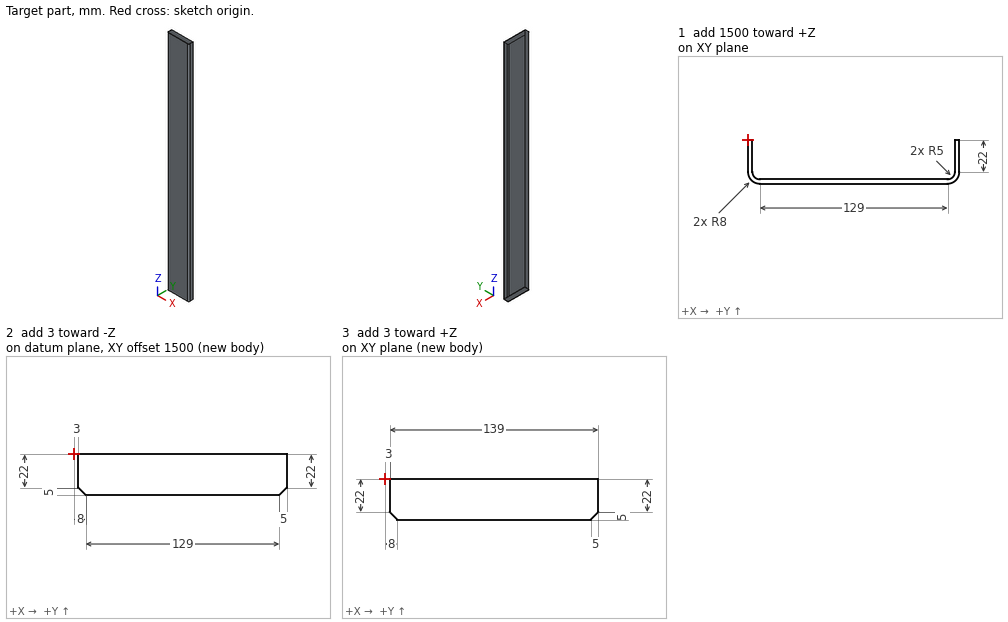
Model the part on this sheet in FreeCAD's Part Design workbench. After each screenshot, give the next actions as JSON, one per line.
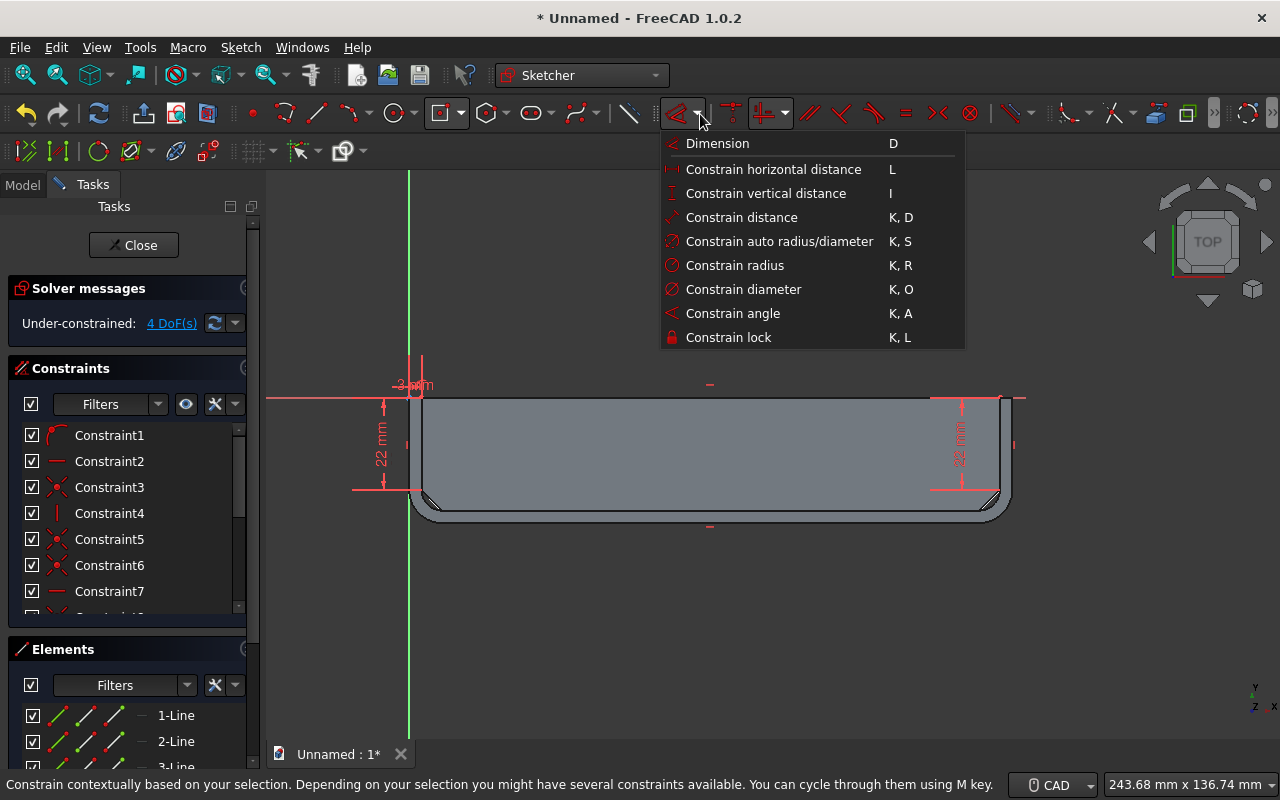
{"action": "left_click", "coordinate": [813, 169]}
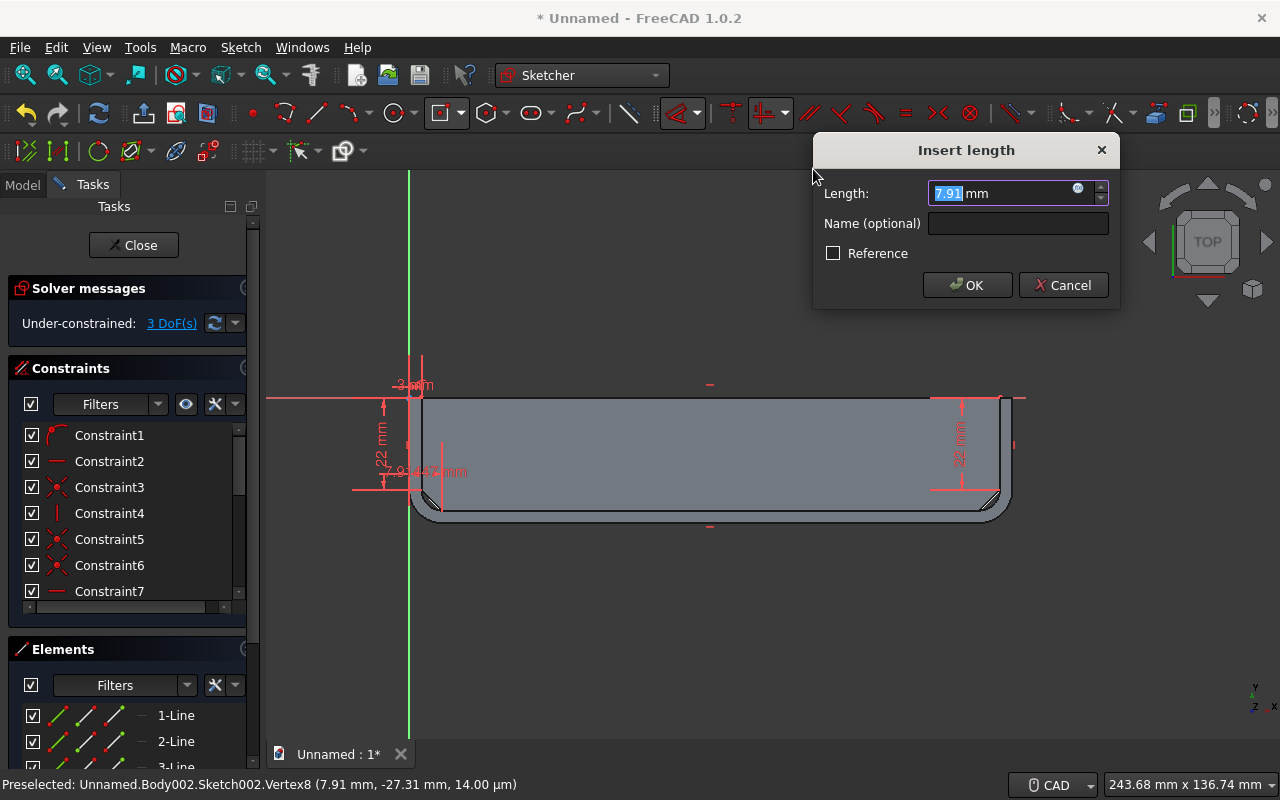
{"action": "type", "text": "8"}
{"action": "key", "text": "Return"}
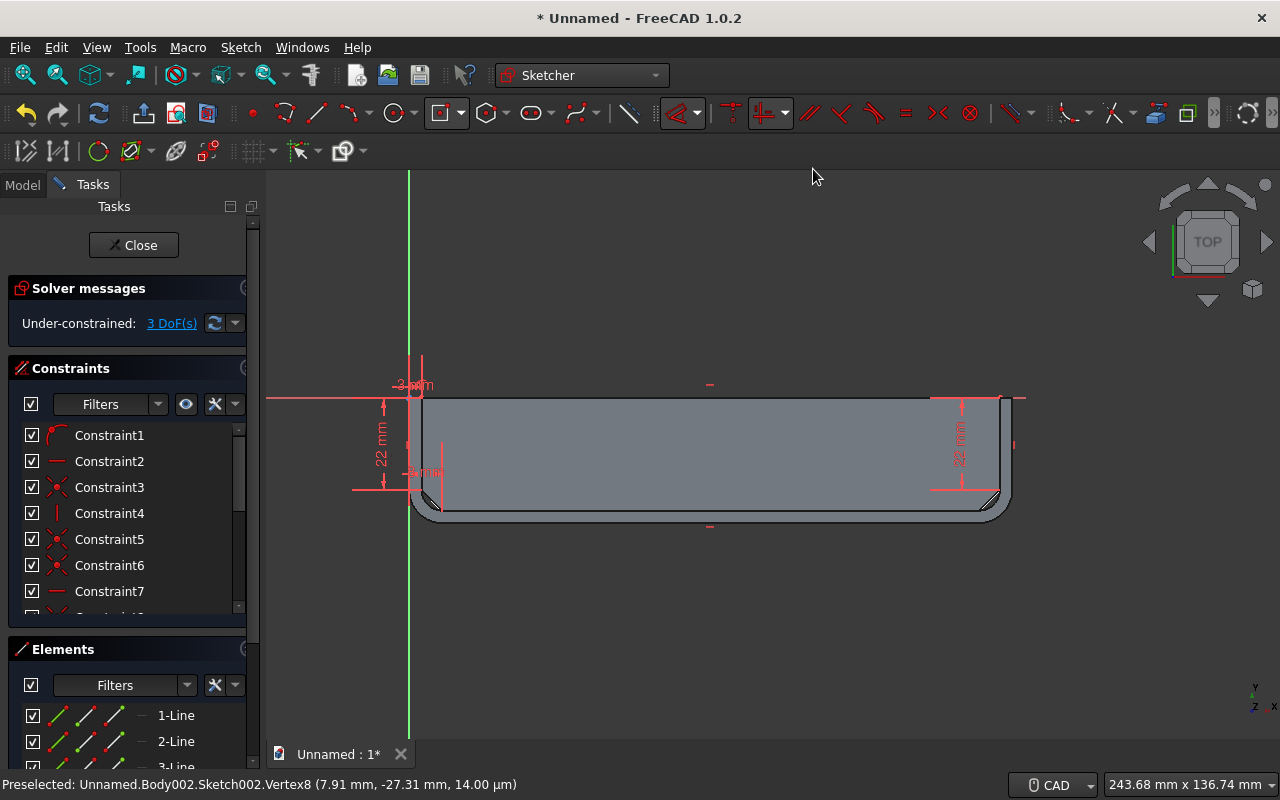
{"action": "scroll", "coordinate": [994, 497], "scroll_direction": "up", "scroll_amount": 4}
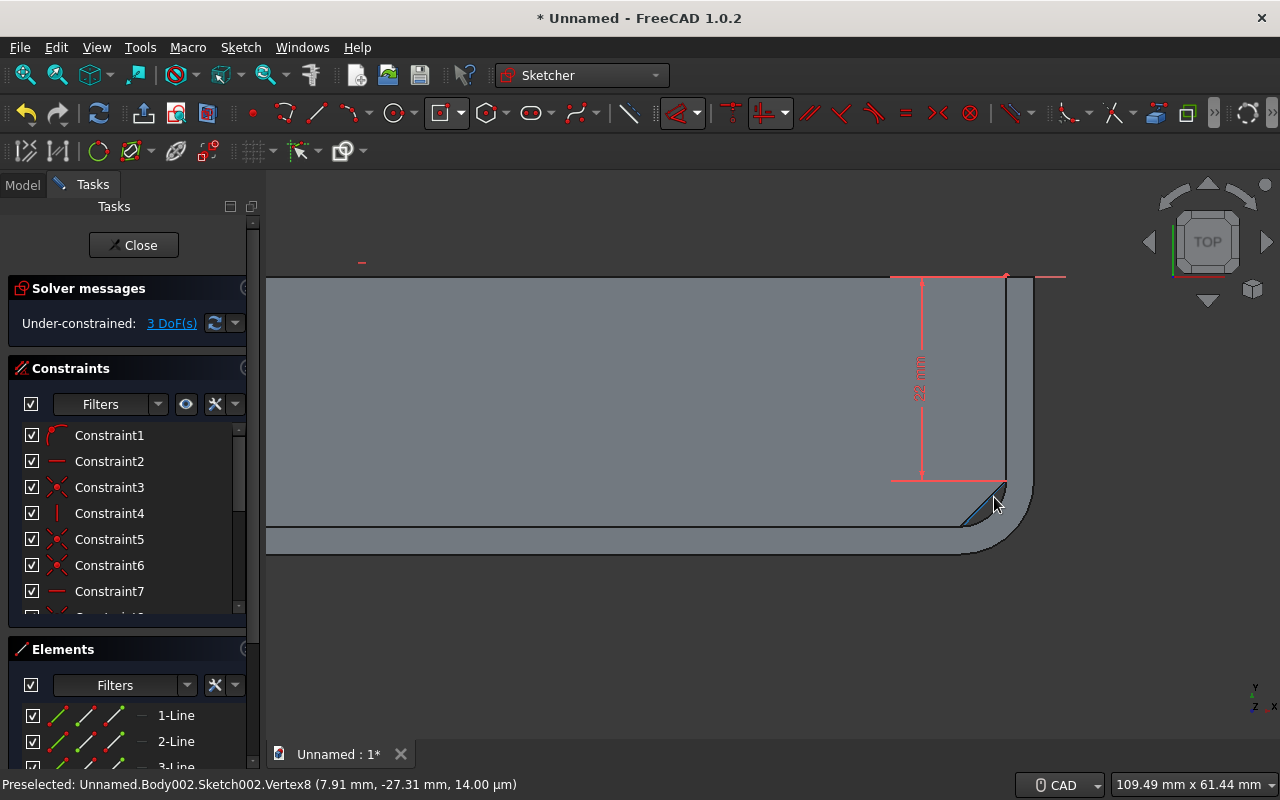
{"action": "left_click", "coordinate": [992, 495]}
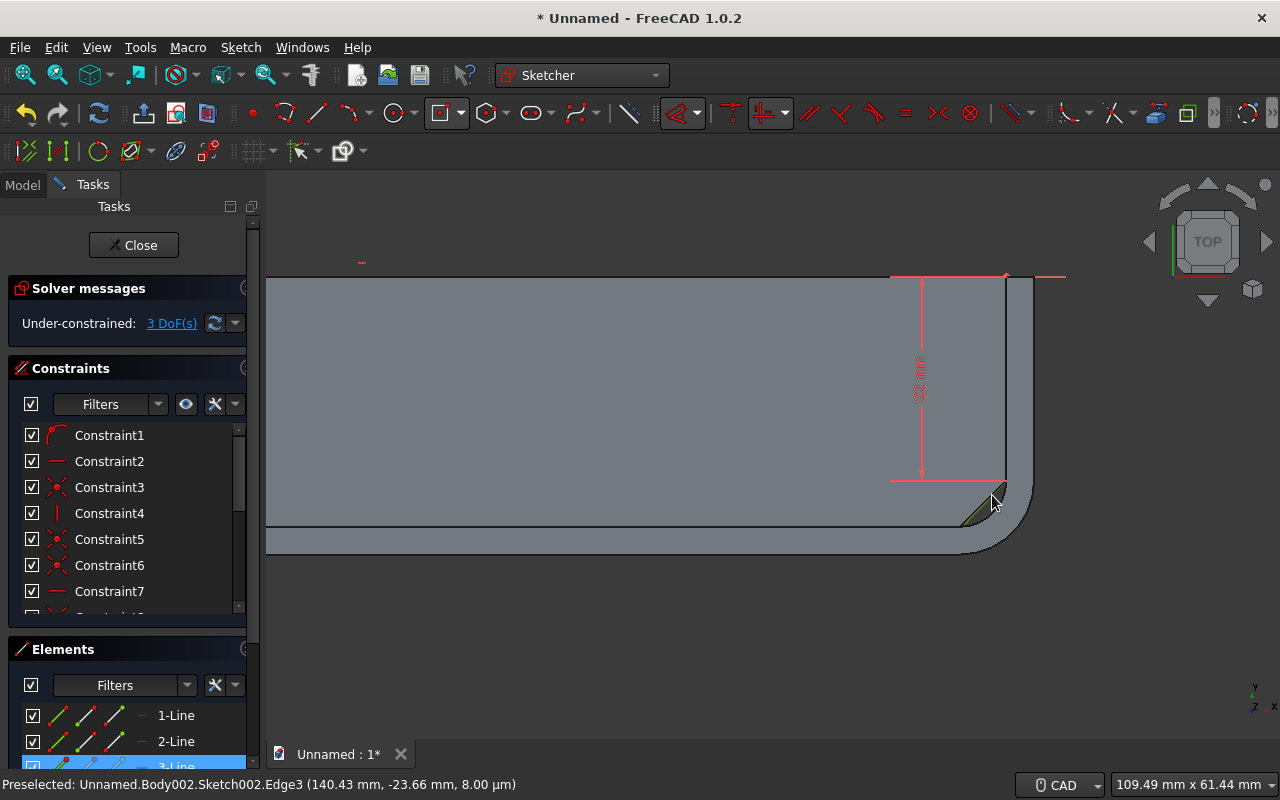
{"action": "key", "text": "l"}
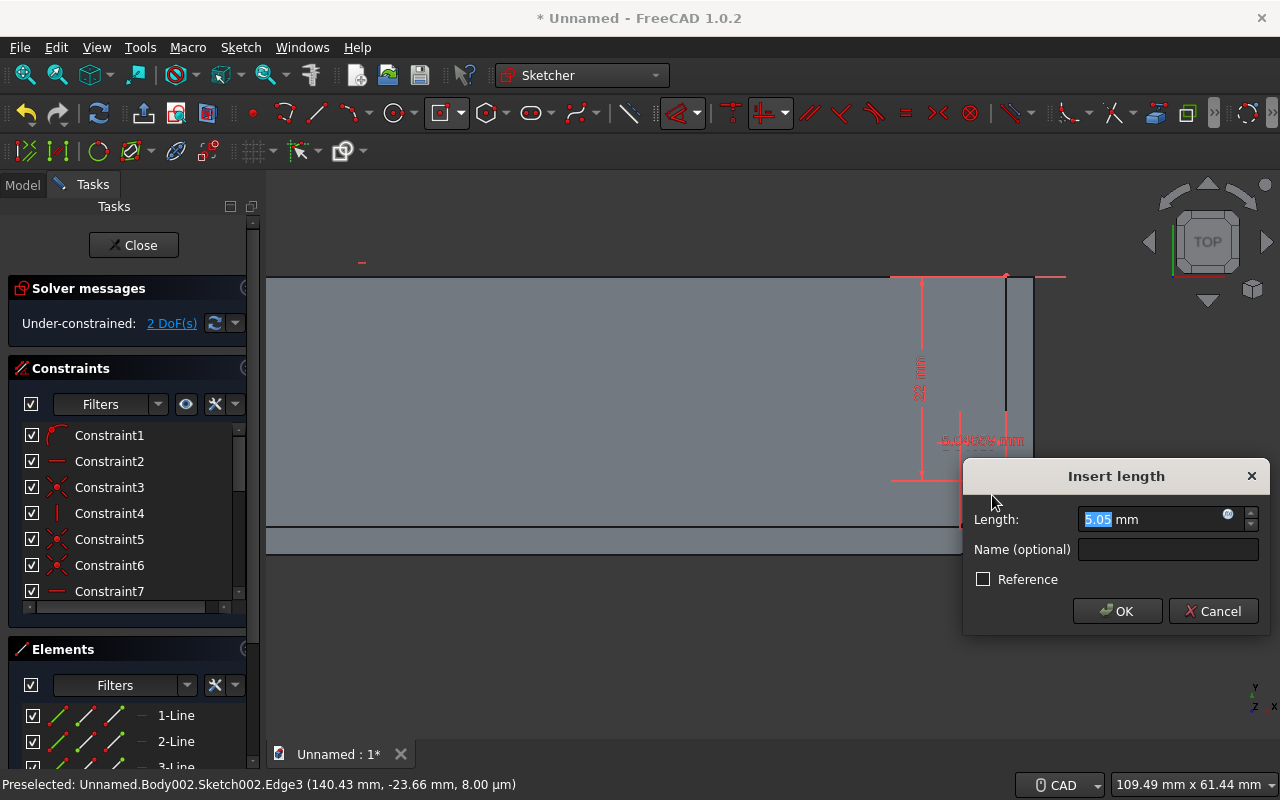
{"action": "type", "text": "5"}
{"action": "key", "text": "Return"}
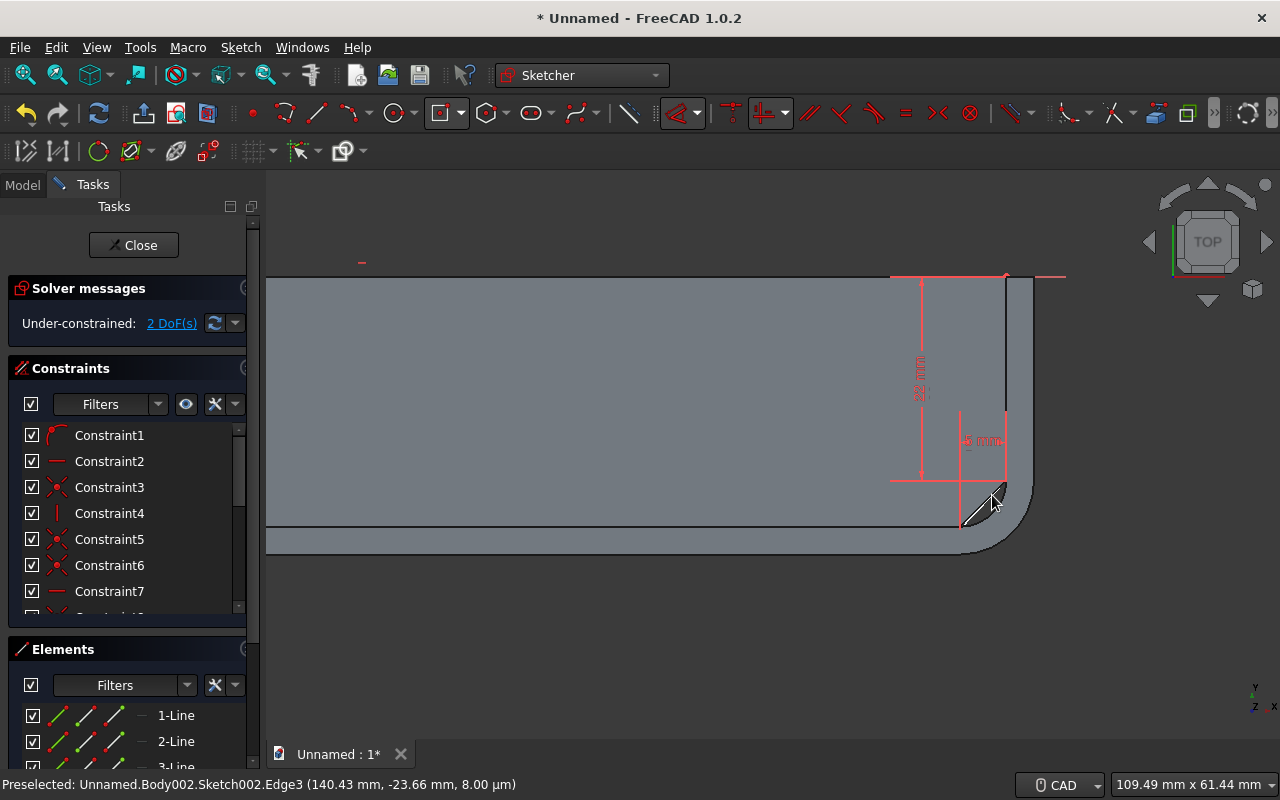
{"action": "left_click", "coordinate": [992, 495]}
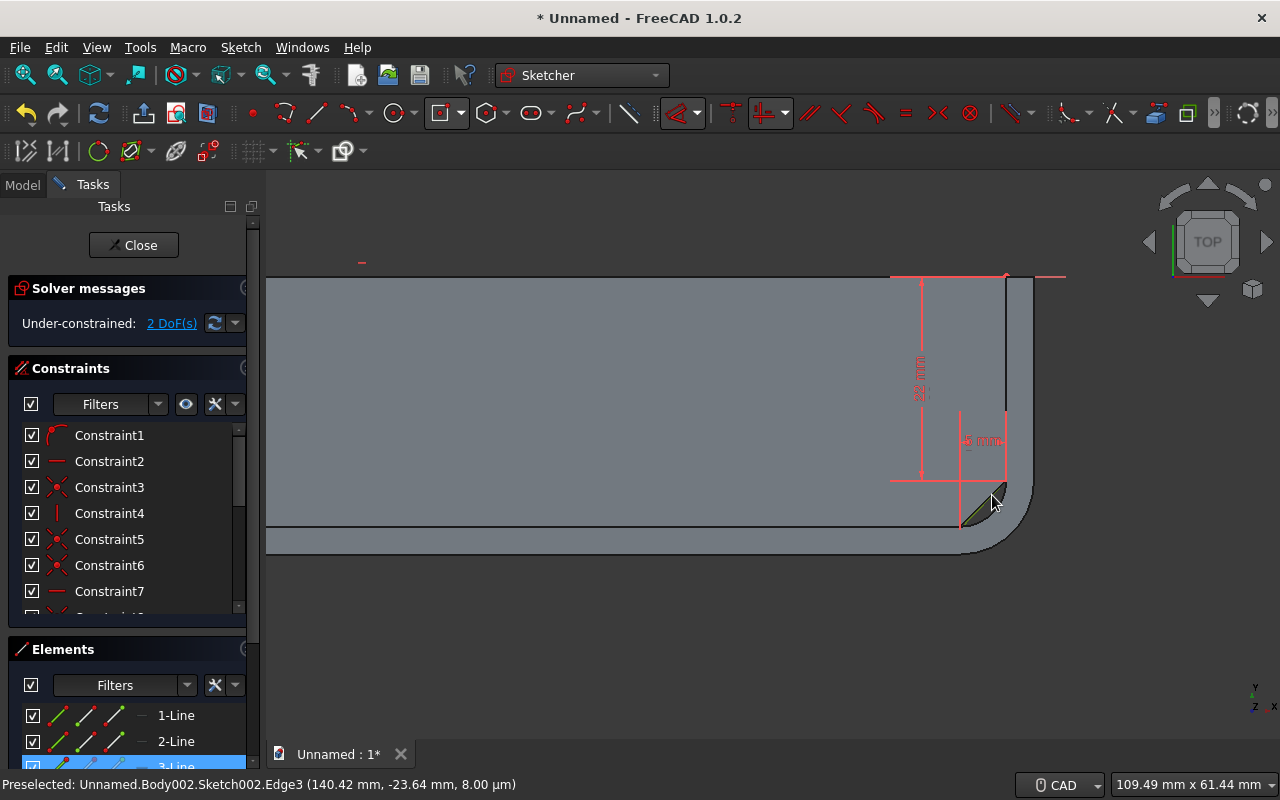
{"action": "key", "text": "i"}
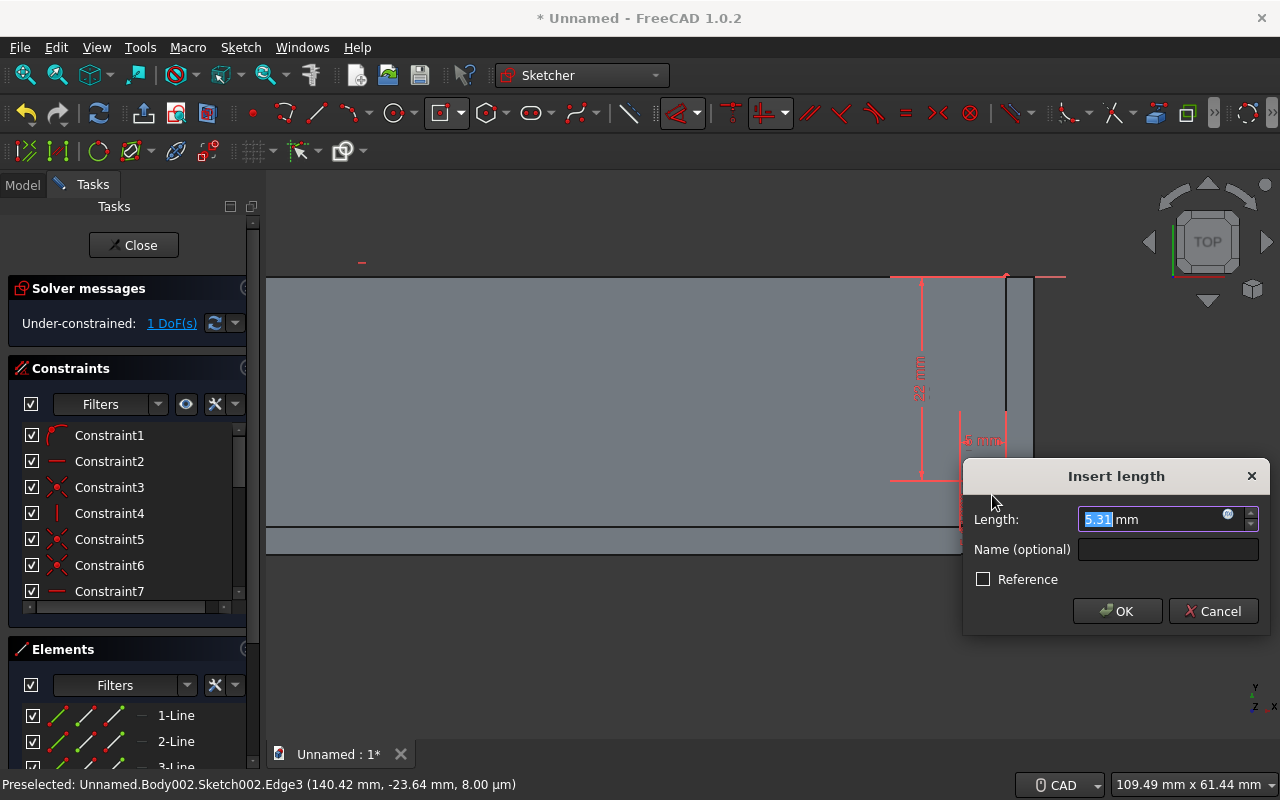
{"action": "type", "text": "5"}
{"action": "key", "text": "Return"}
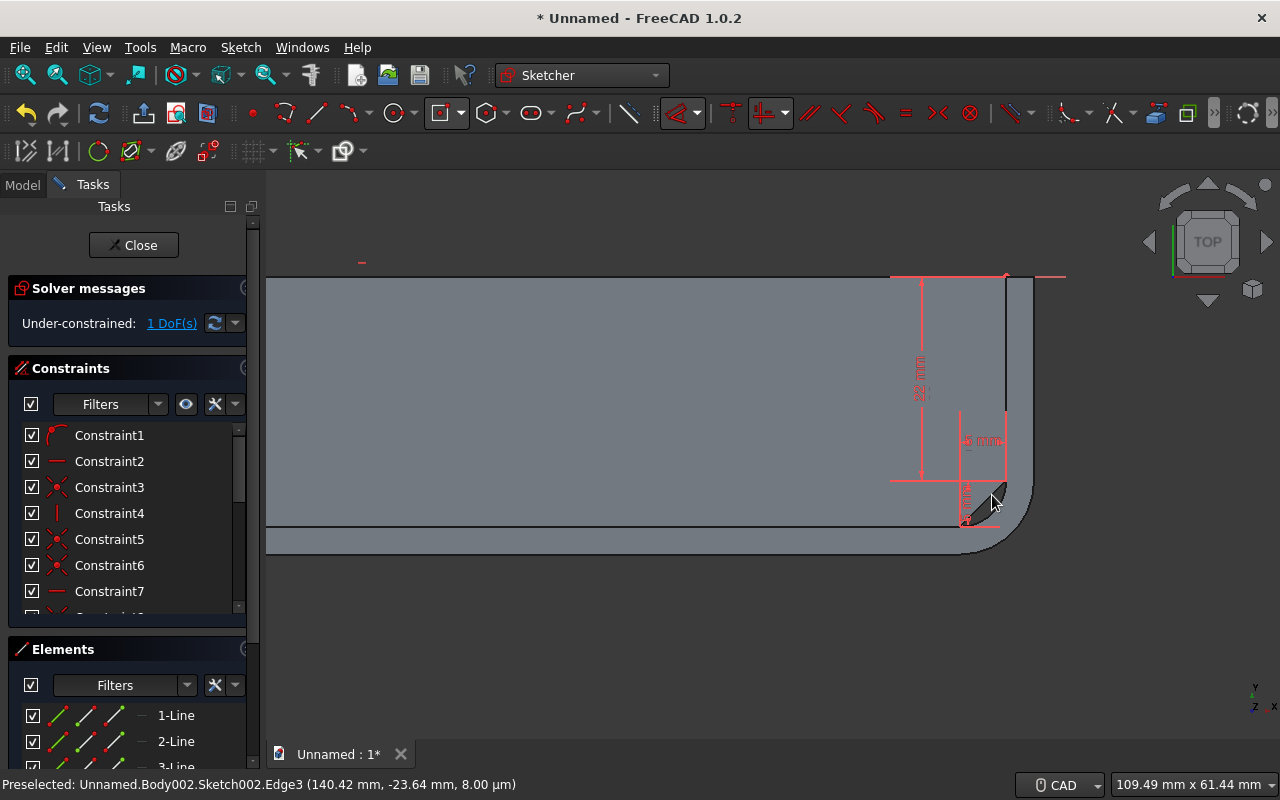
{"action": "left_click", "coordinate": [620, 277]}